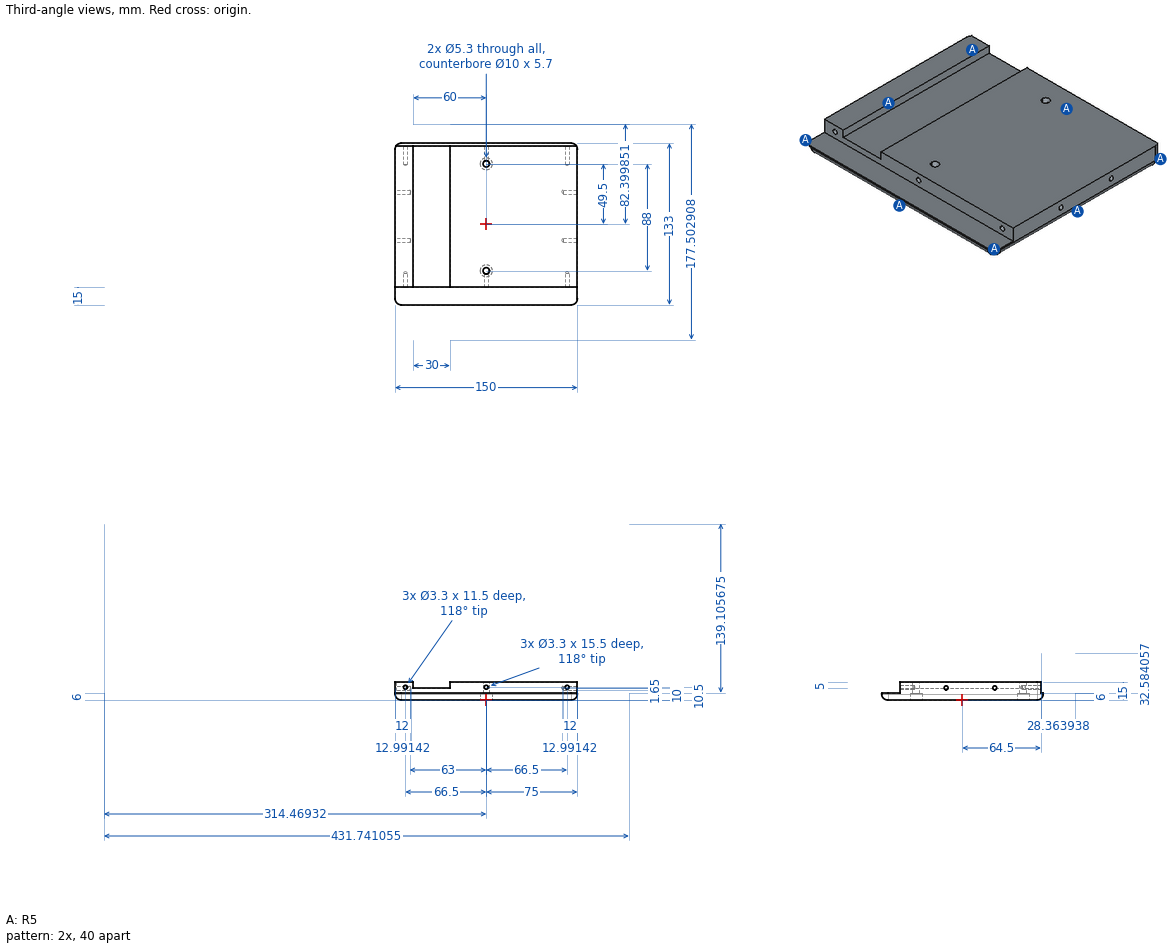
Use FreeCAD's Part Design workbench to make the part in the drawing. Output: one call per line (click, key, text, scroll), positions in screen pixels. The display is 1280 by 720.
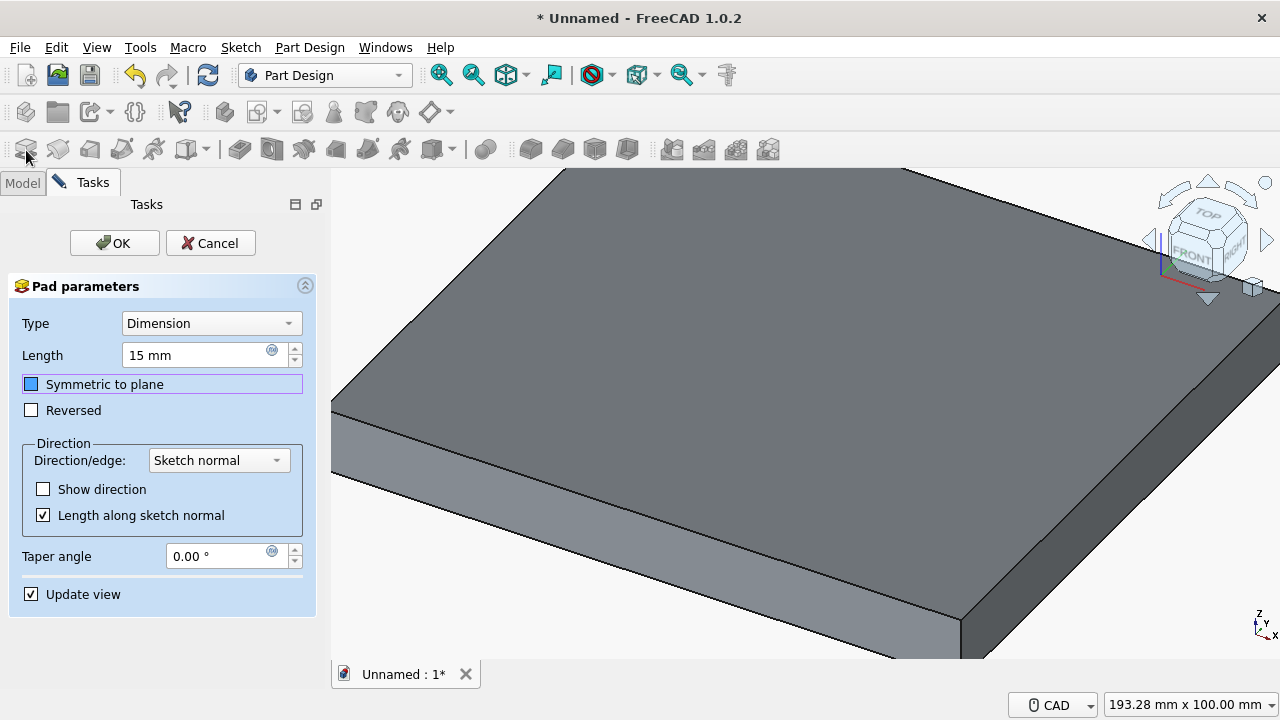
click(115, 243)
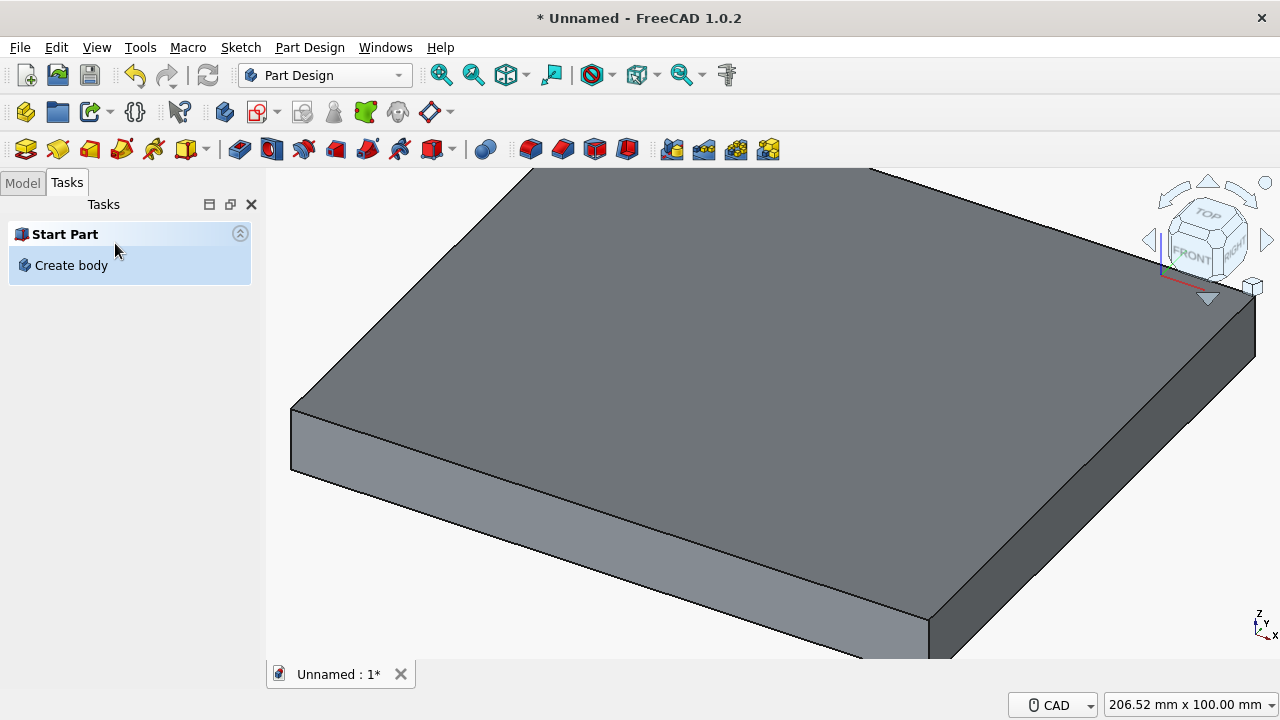
click(442, 76)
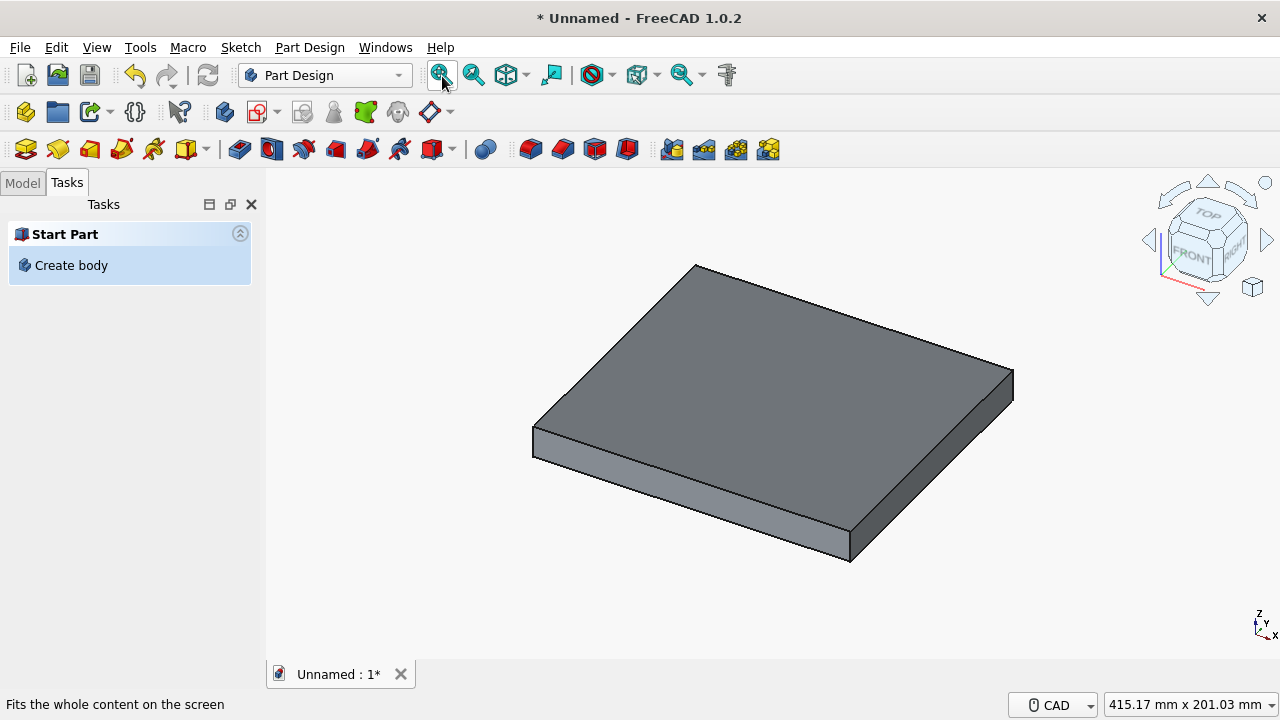
click(1001, 396)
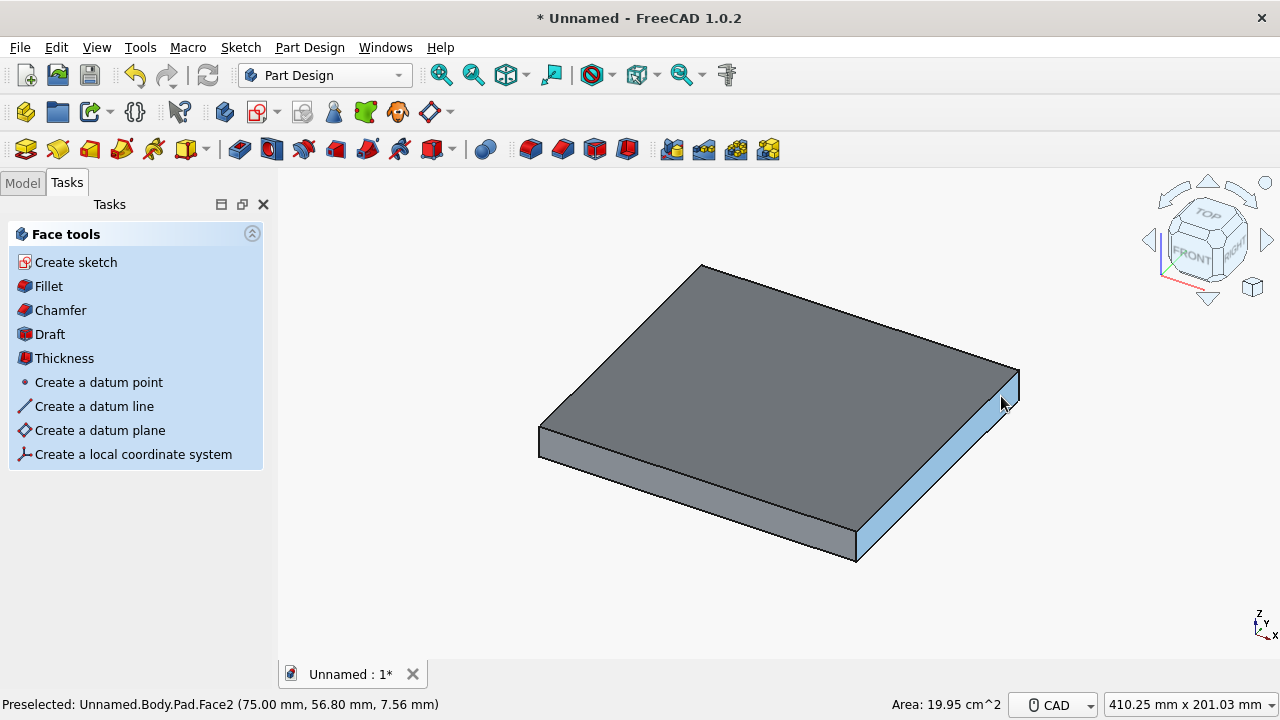
click(258, 112)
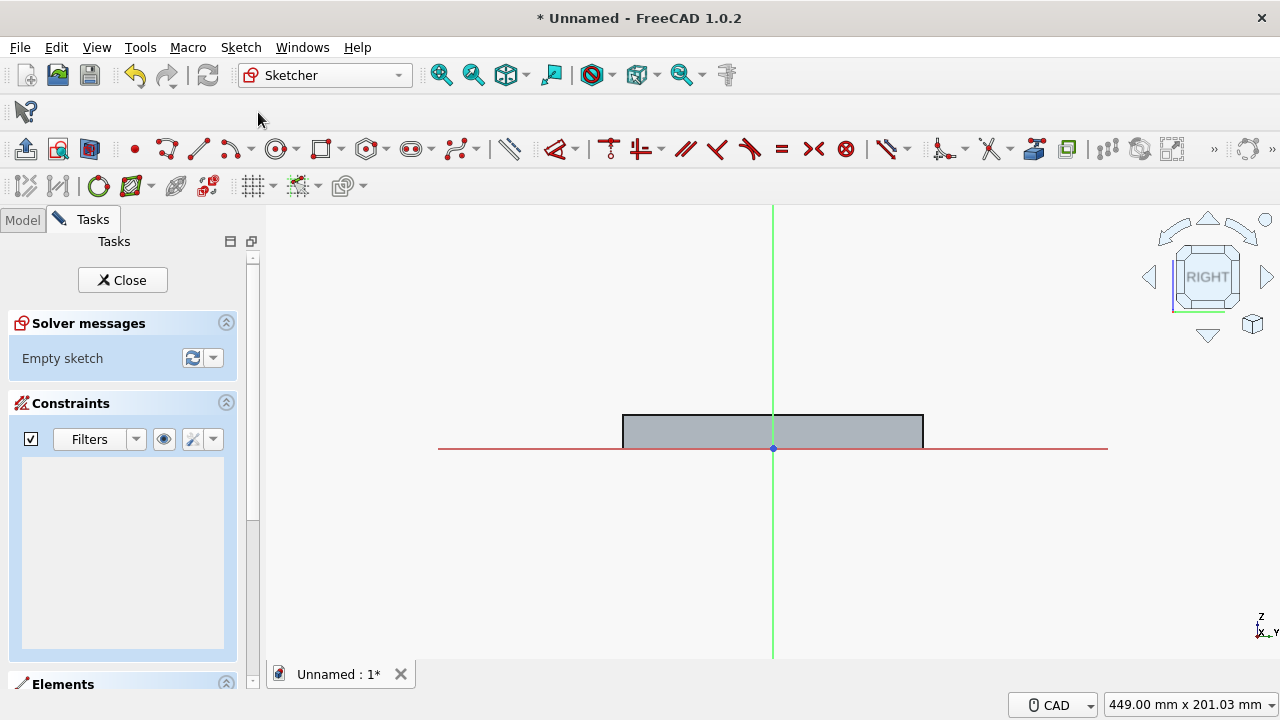
scroll(1031, 388, up, 7)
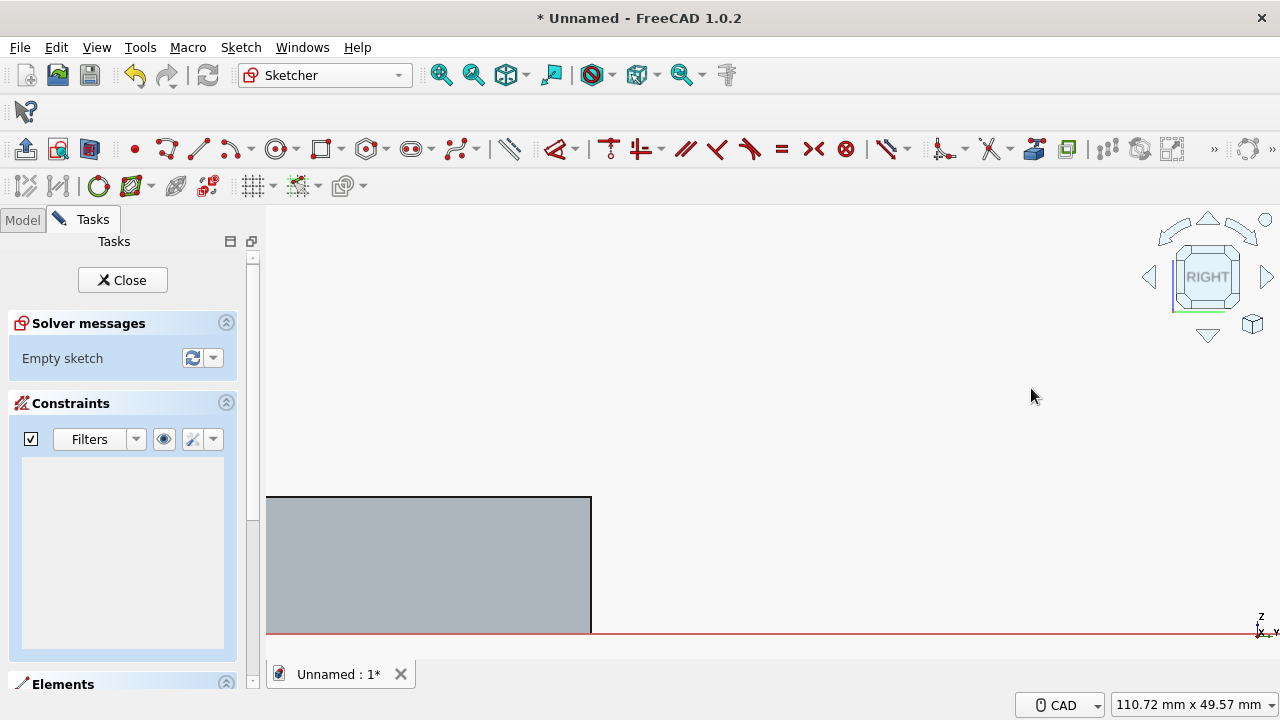
click(322, 150)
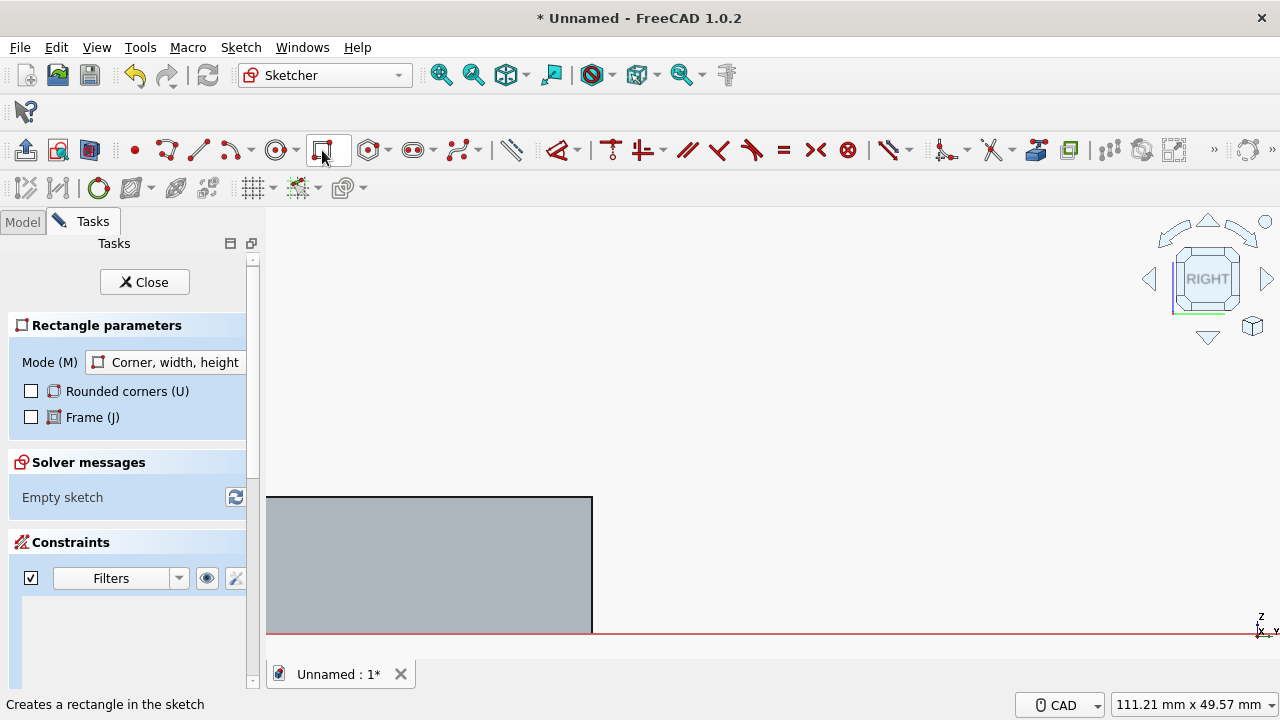
click(574, 282)
move(833, 579)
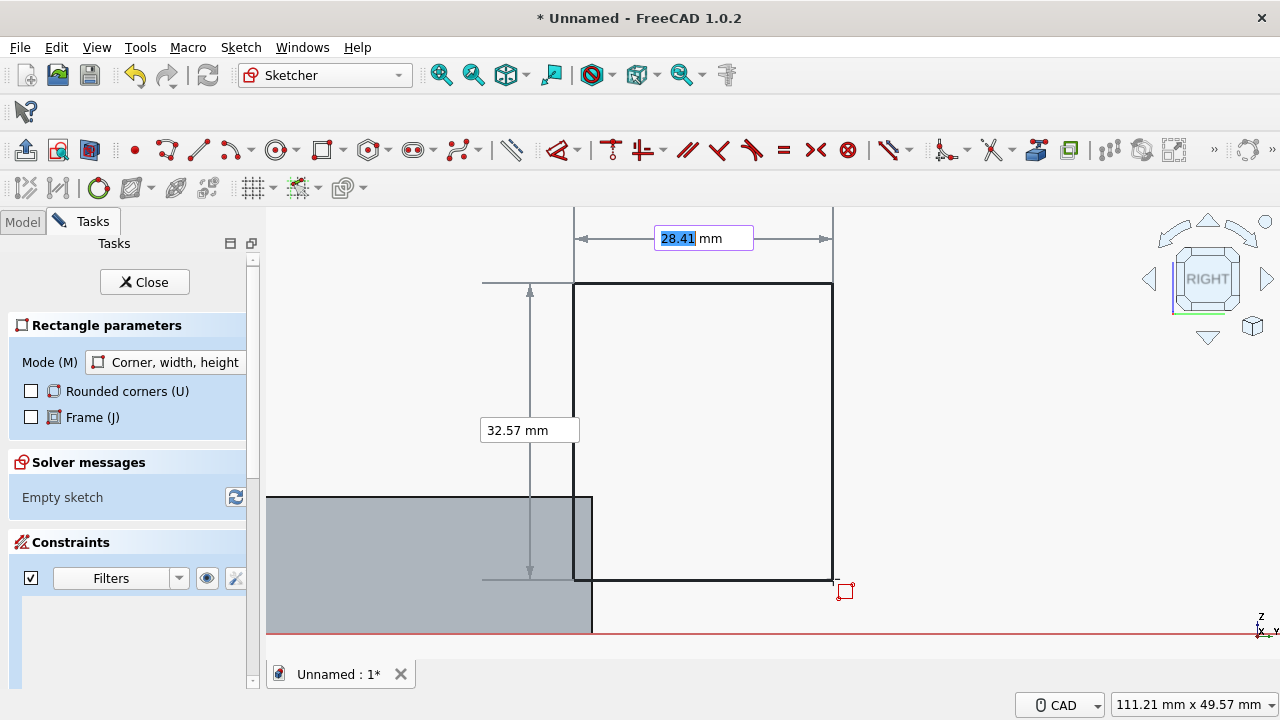
text(28.363938)
key(Tab)
text(32.584057)
key(Return)
key(Escape)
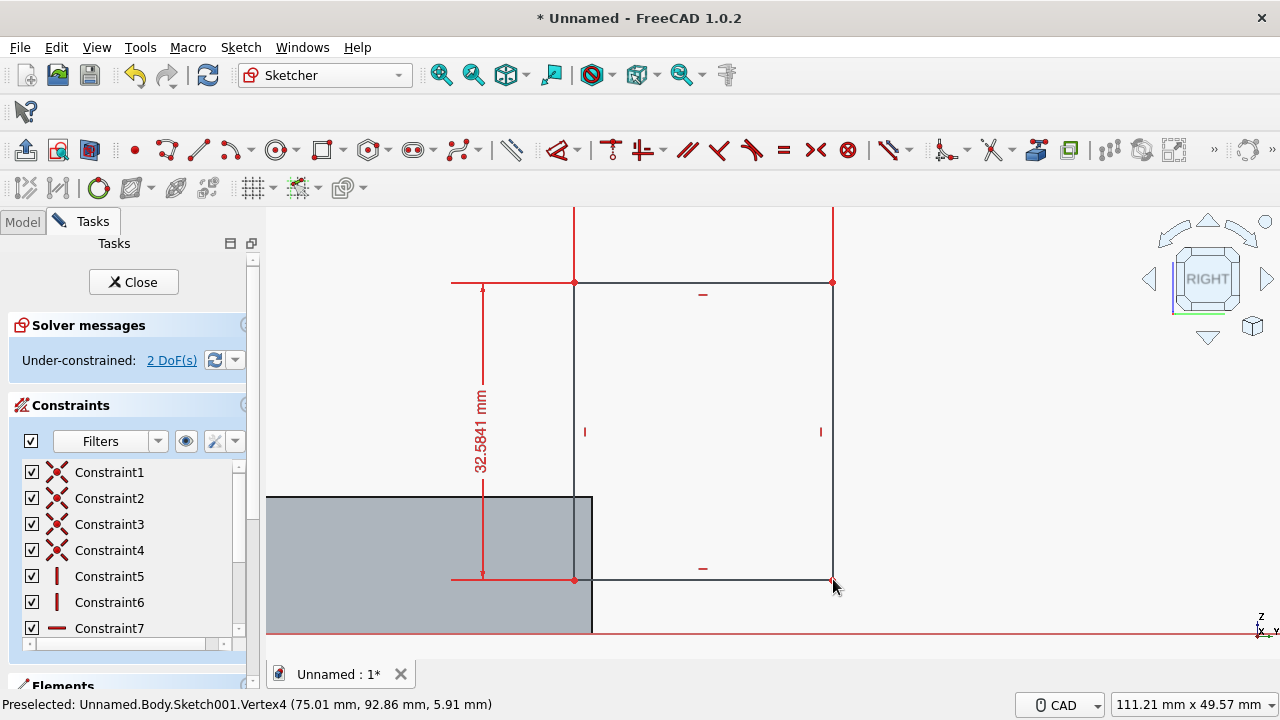
click(558, 150)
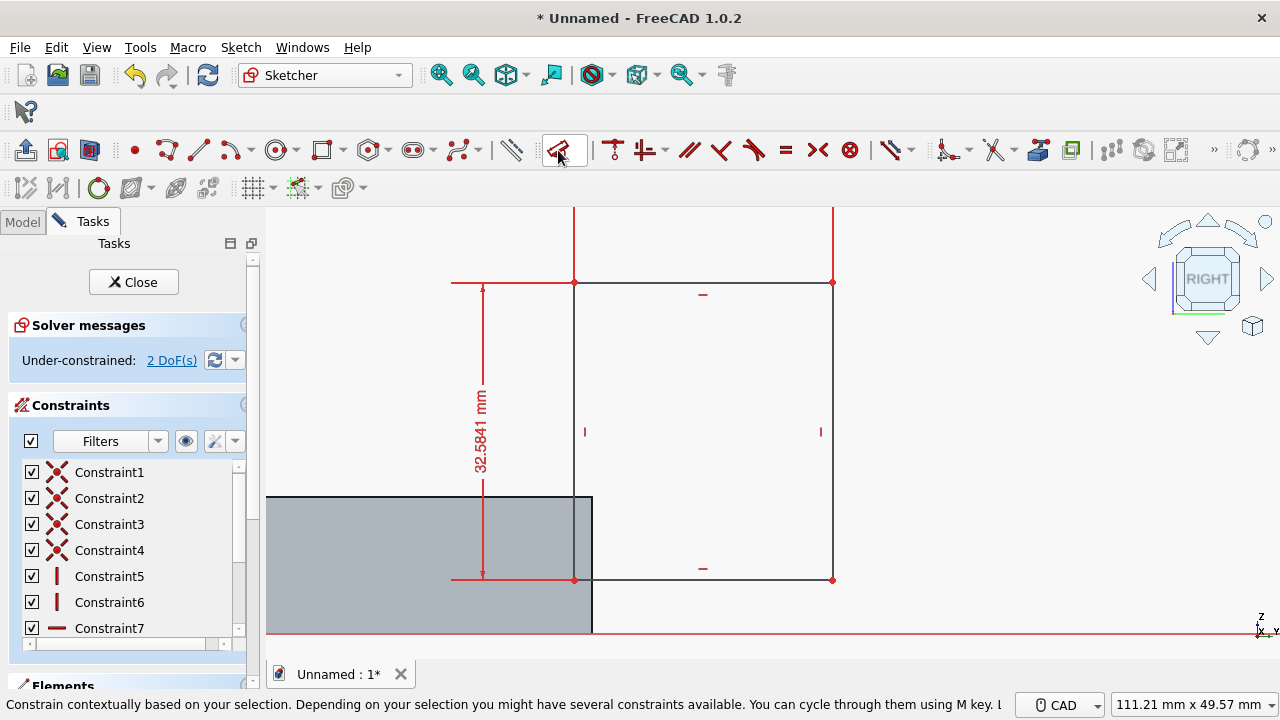
click(574, 580)
click(608, 606)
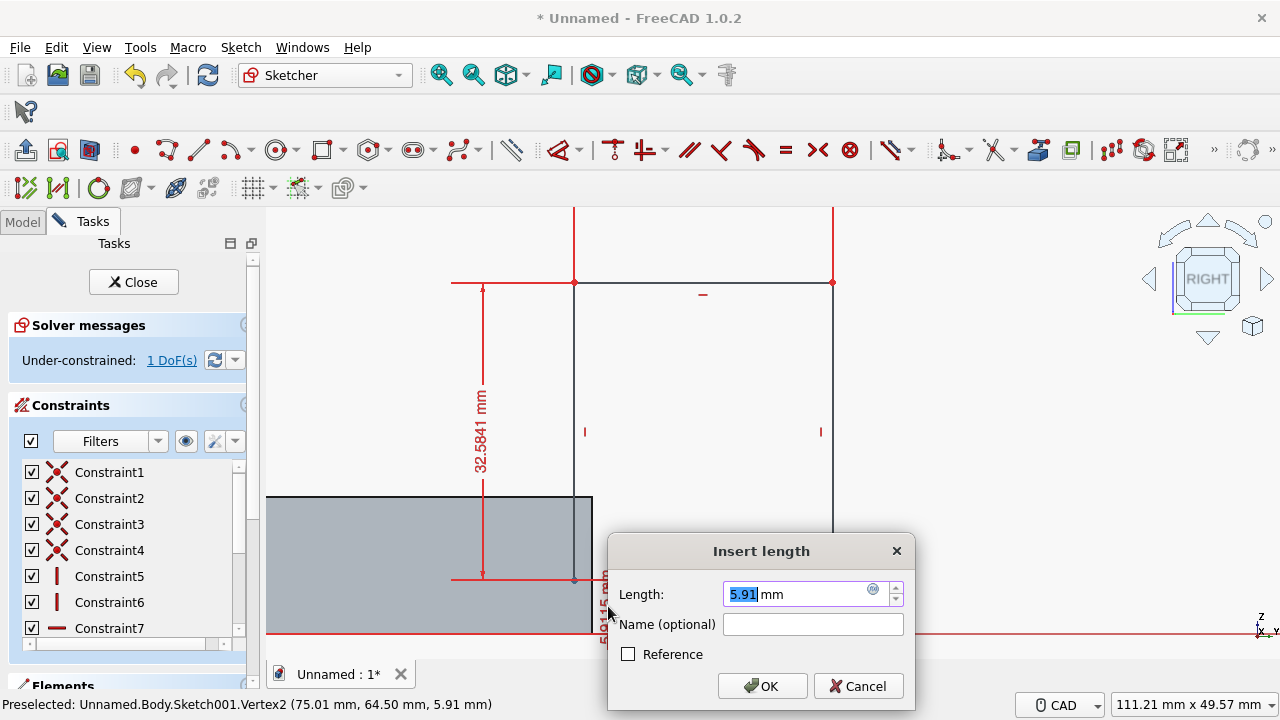
text(6)
key(Return)